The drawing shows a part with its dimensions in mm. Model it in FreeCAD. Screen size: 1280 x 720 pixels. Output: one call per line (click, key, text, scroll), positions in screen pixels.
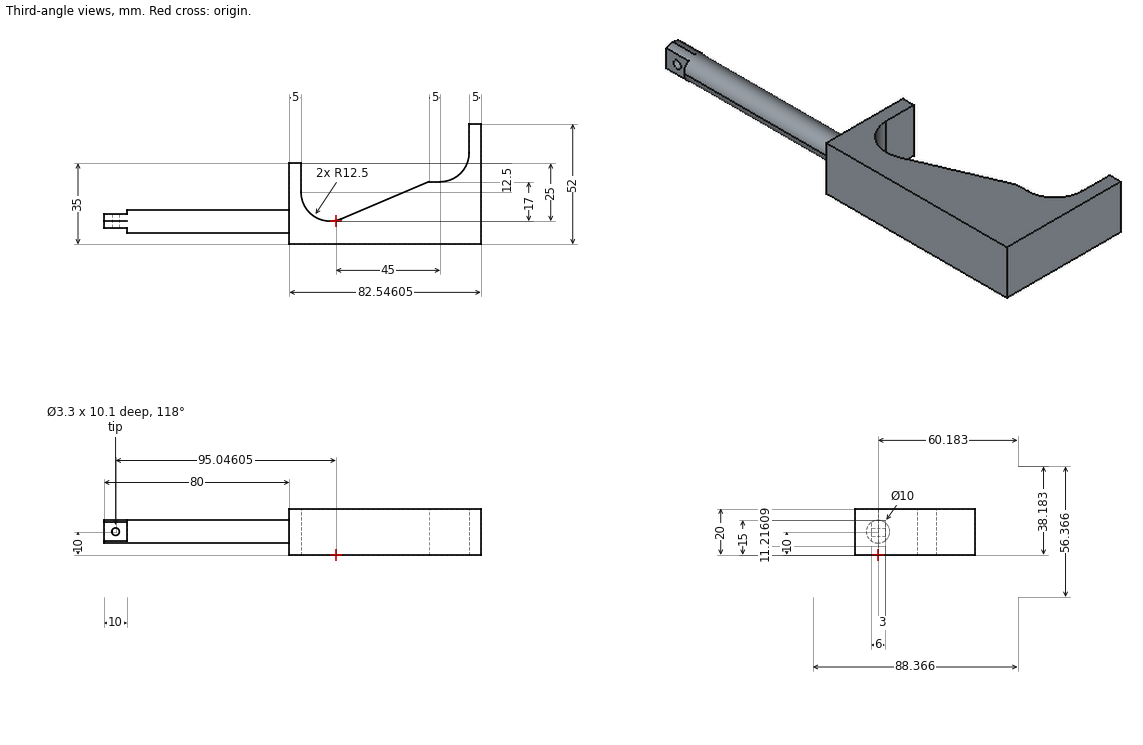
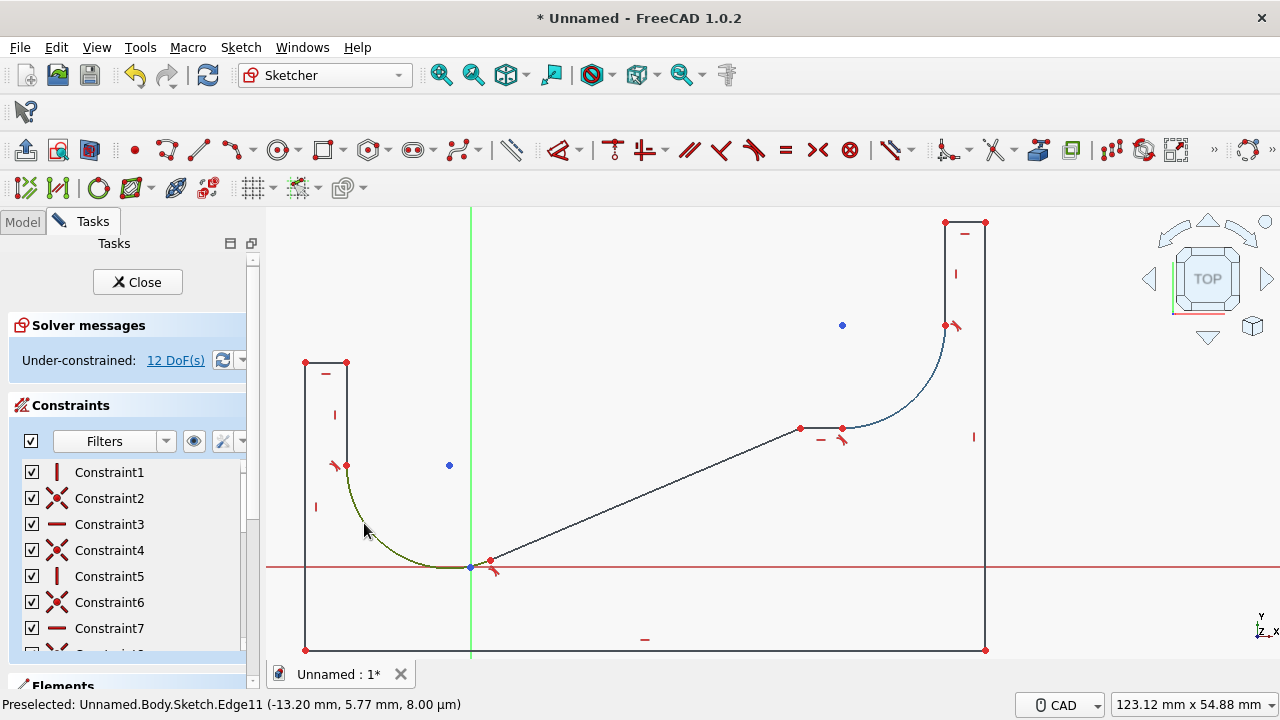
click(786, 150)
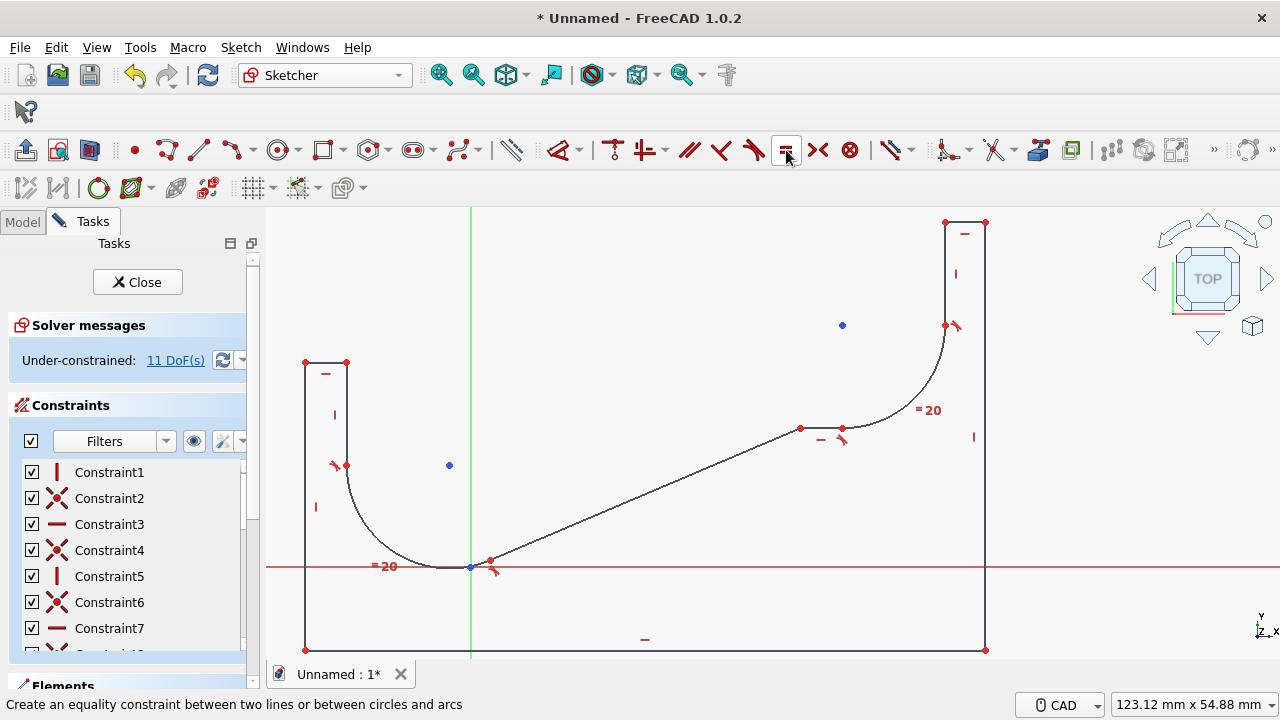
click(558, 150)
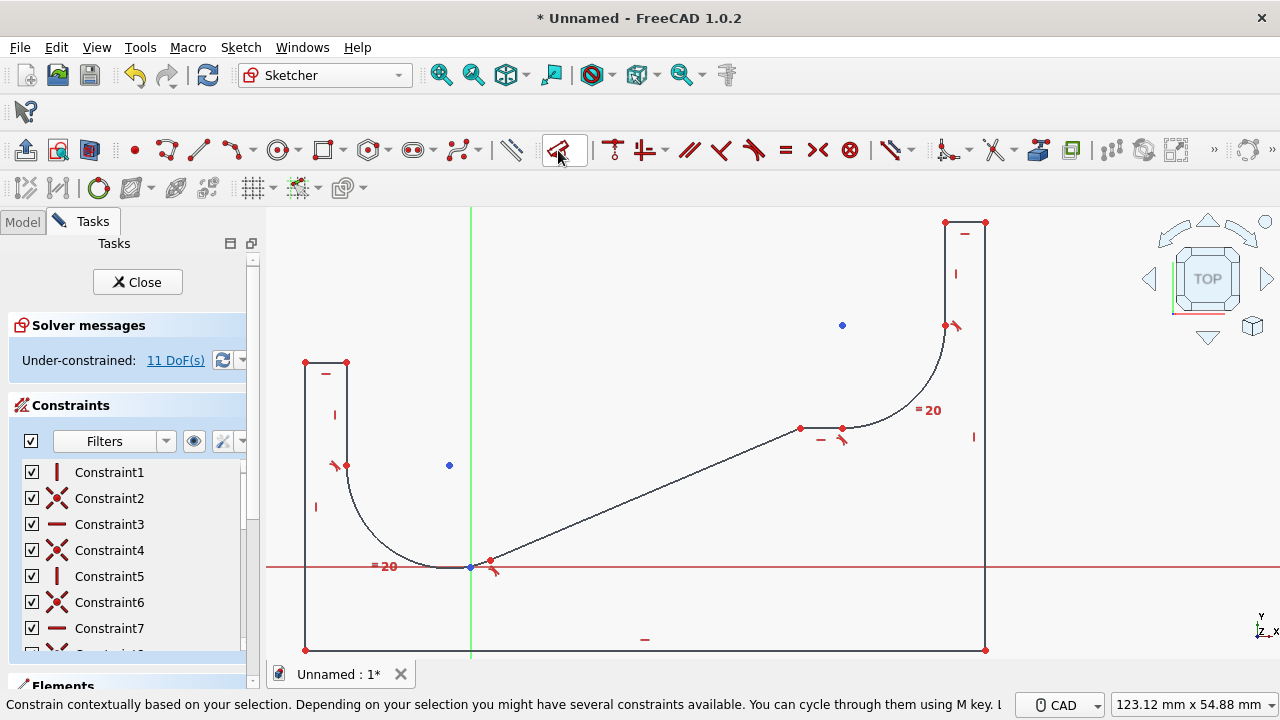
click(889, 417)
click(904, 445)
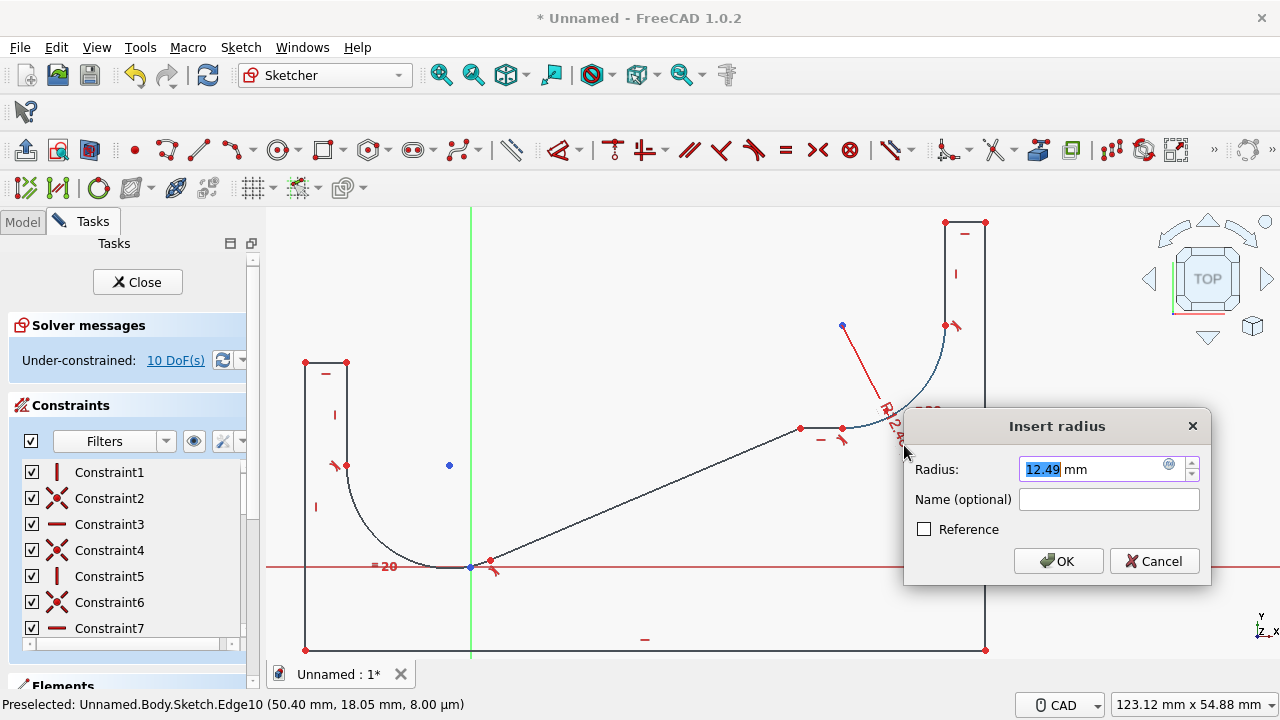
text(12.5)
key(Return)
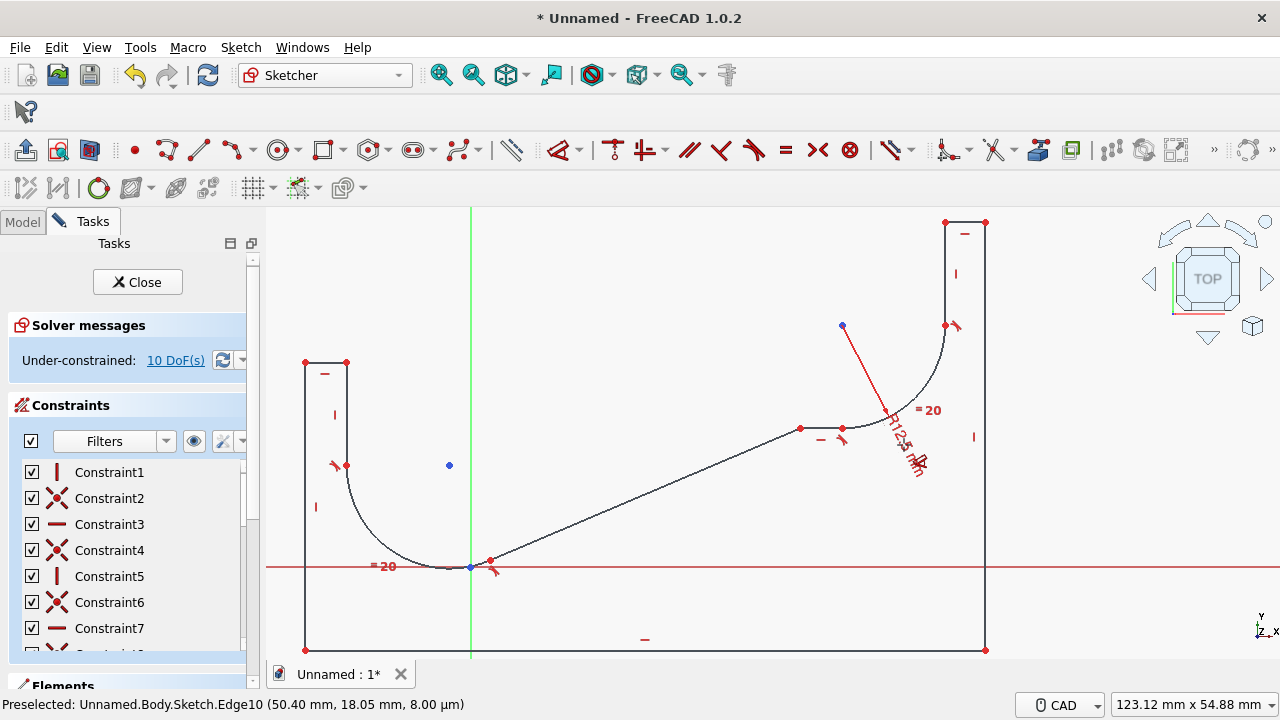
click(334, 363)
click(326, 329)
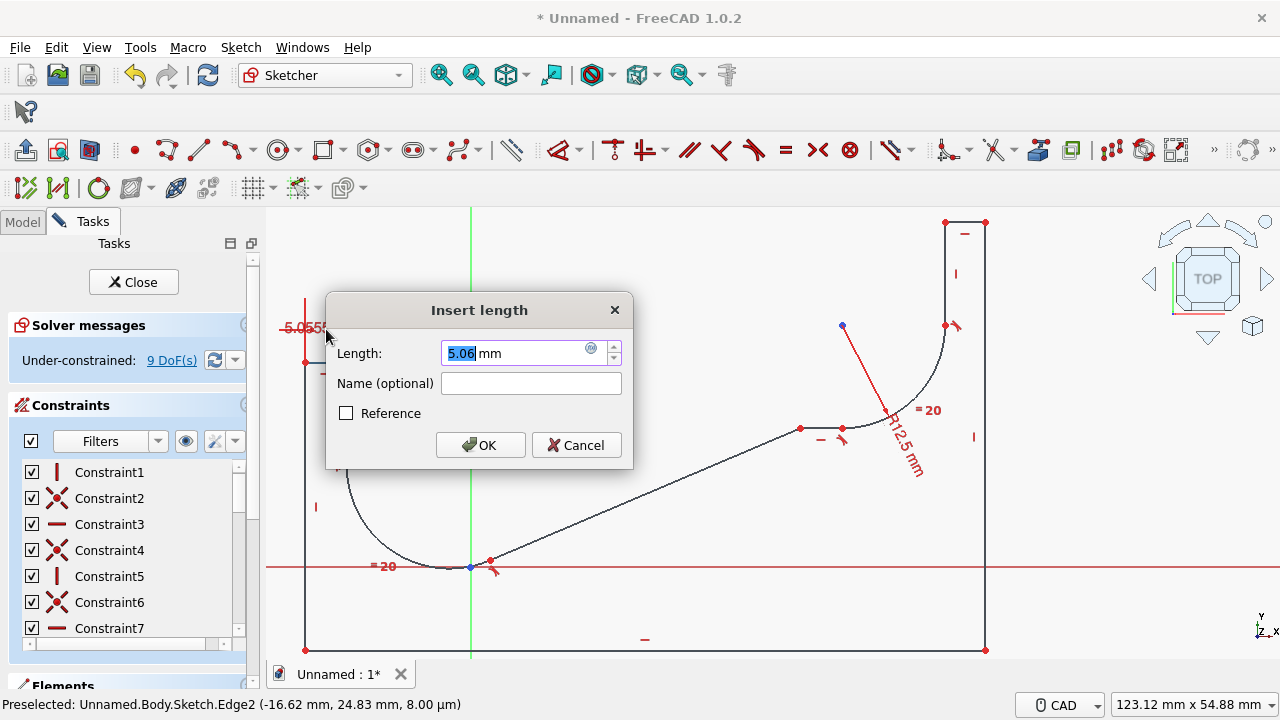
text(5)
key(Return)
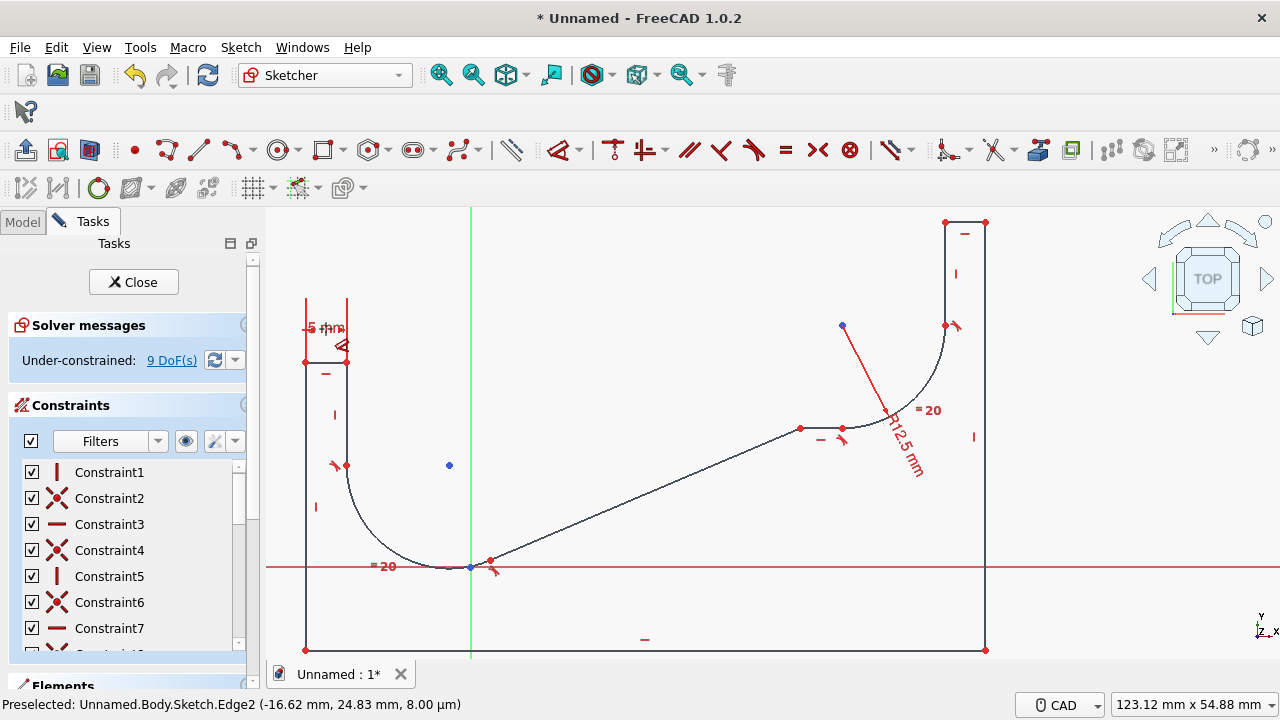
scroll(824, 428, down, 2)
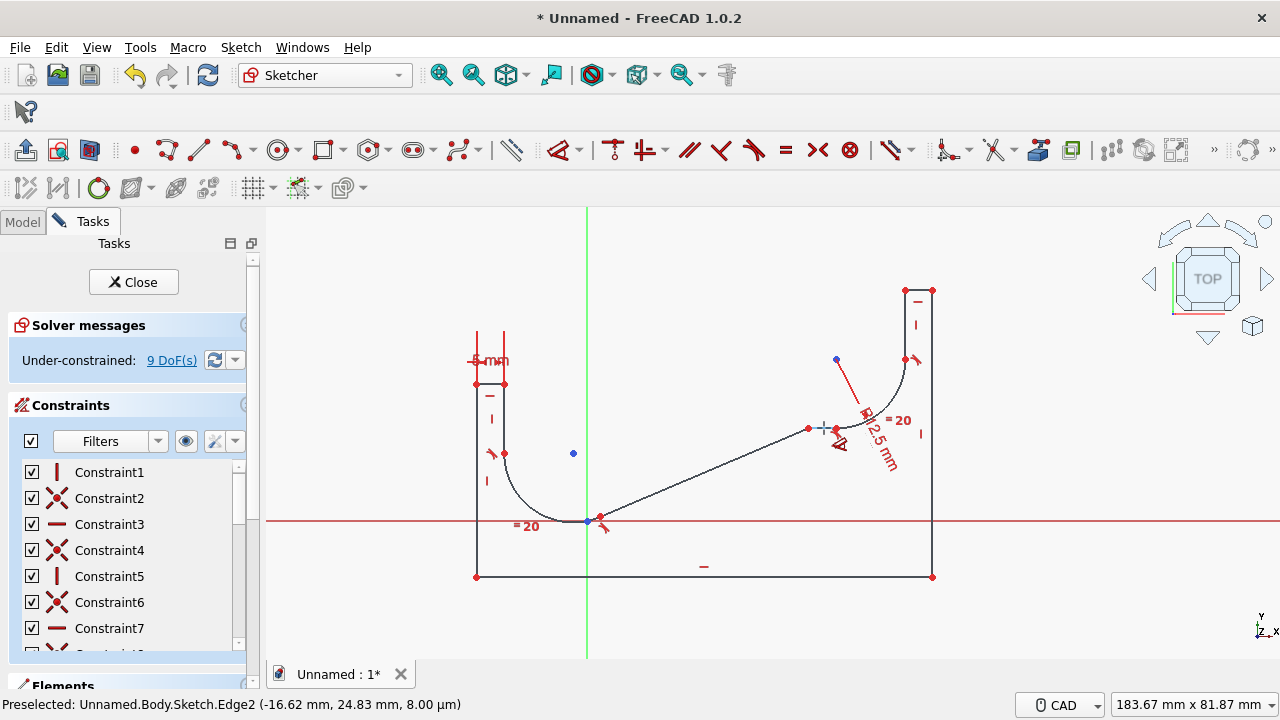
scroll(924, 290, up, 3)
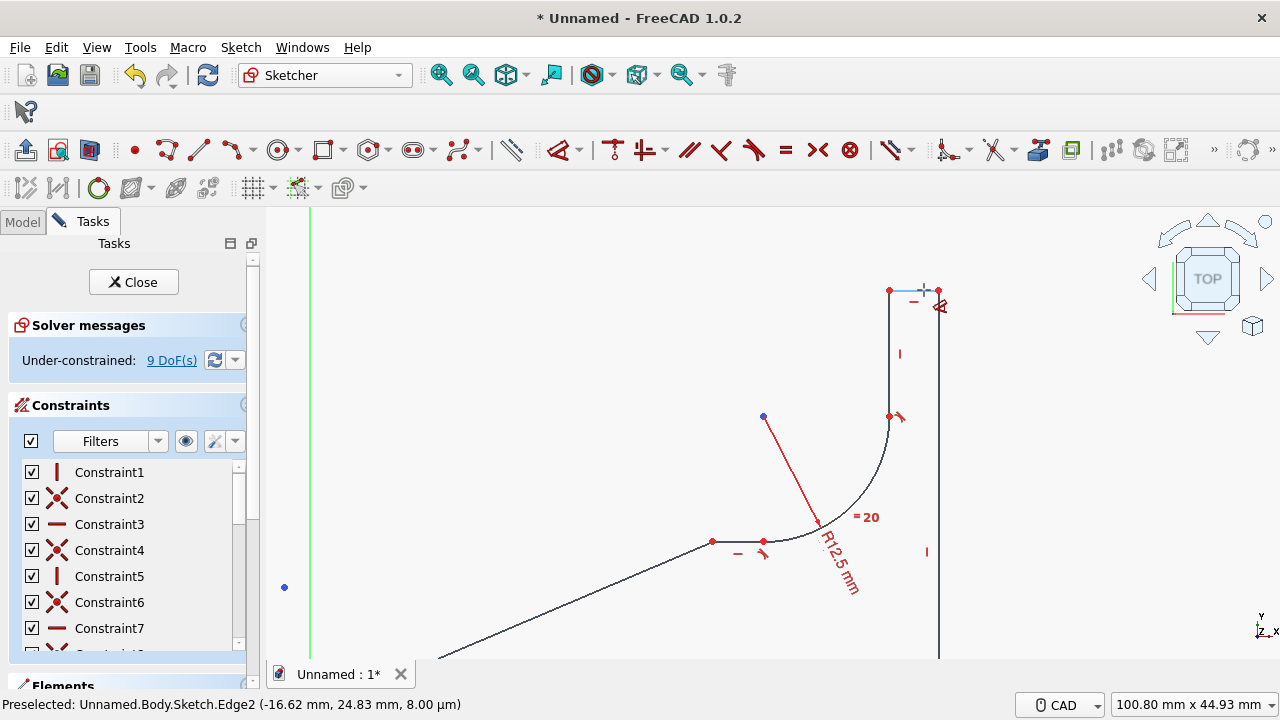
click(924, 291)
click(914, 257)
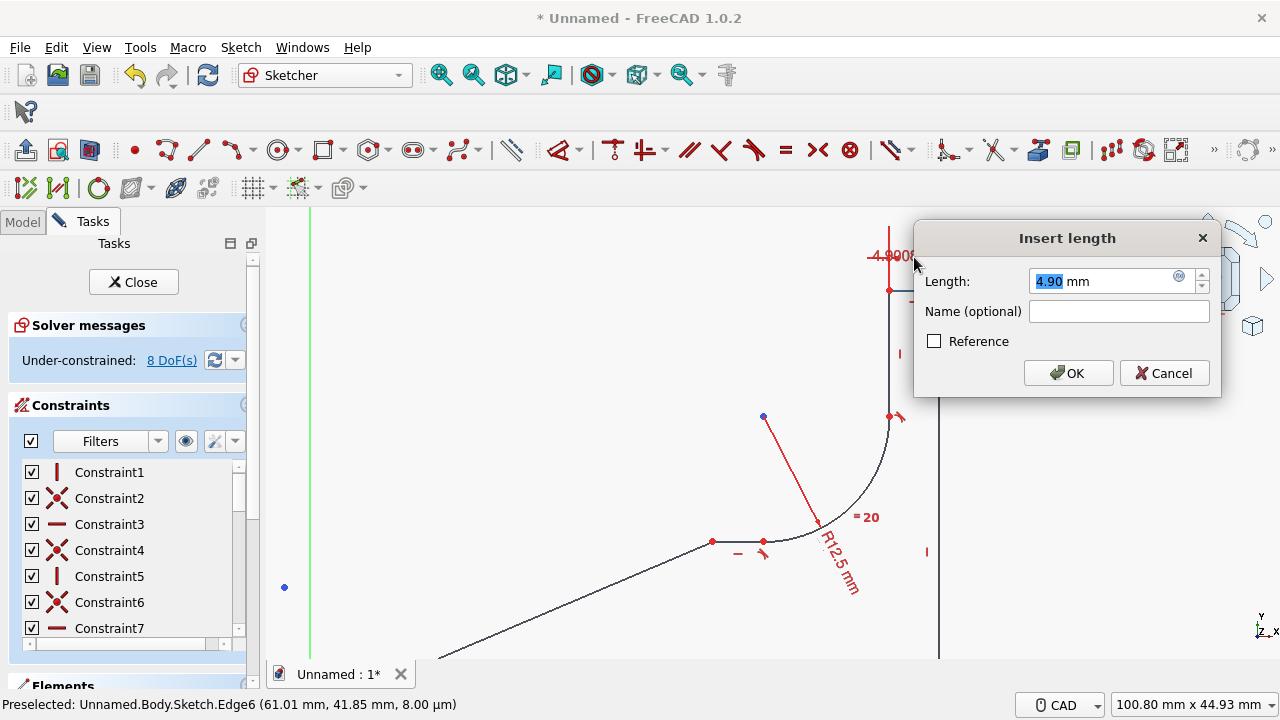
text(5)
key(Return)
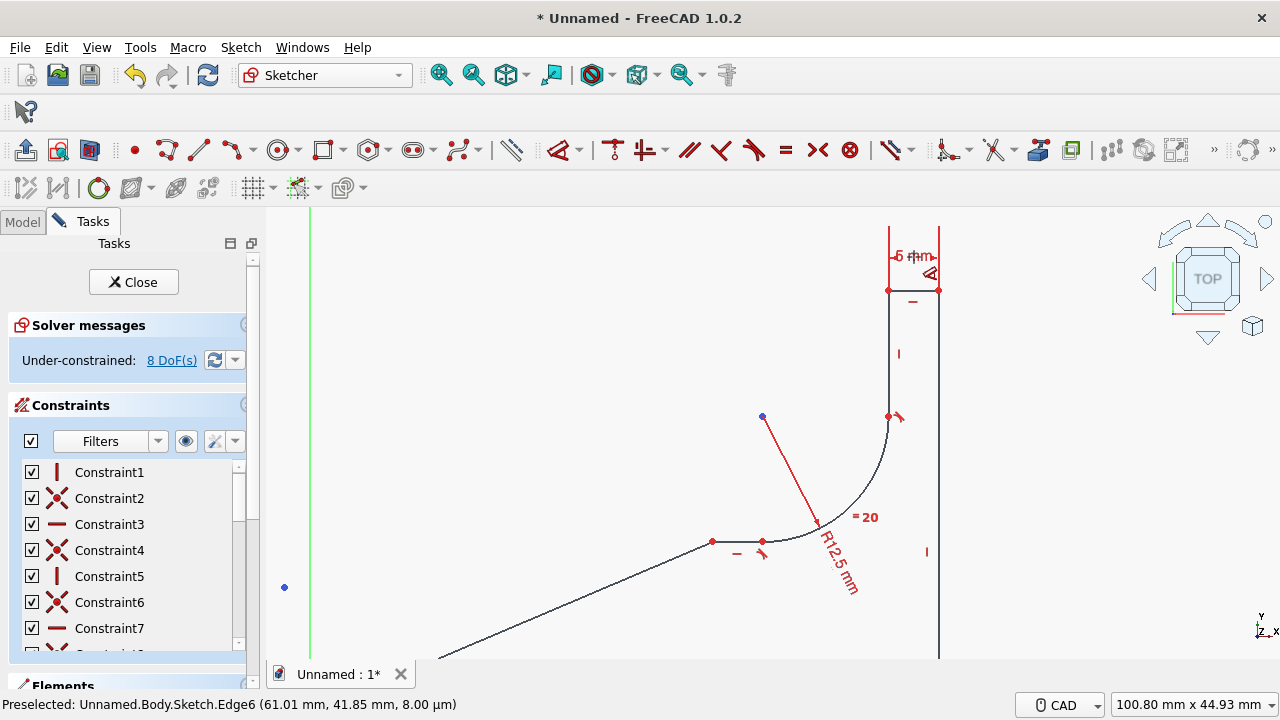
click(748, 542)
click(738, 508)